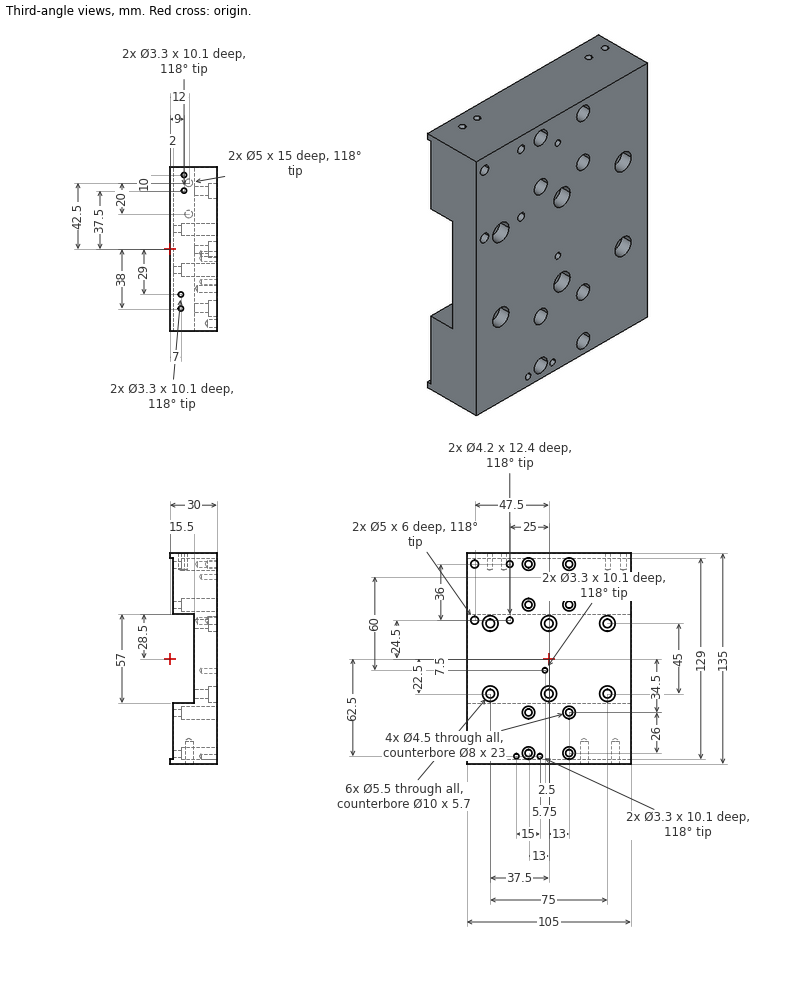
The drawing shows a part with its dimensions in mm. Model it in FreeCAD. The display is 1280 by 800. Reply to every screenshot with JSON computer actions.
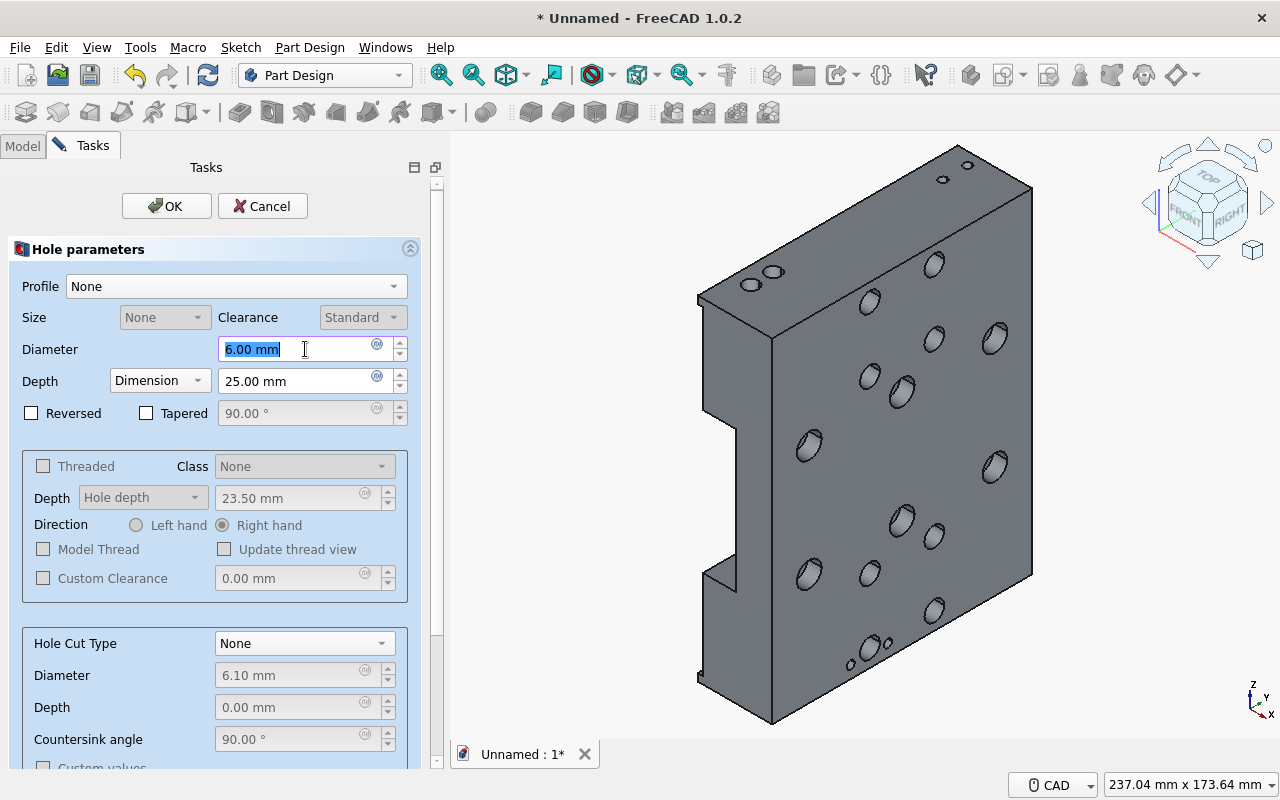
{"action": "type", "text": "3.3"}
{"action": "key", "text": "Tab"}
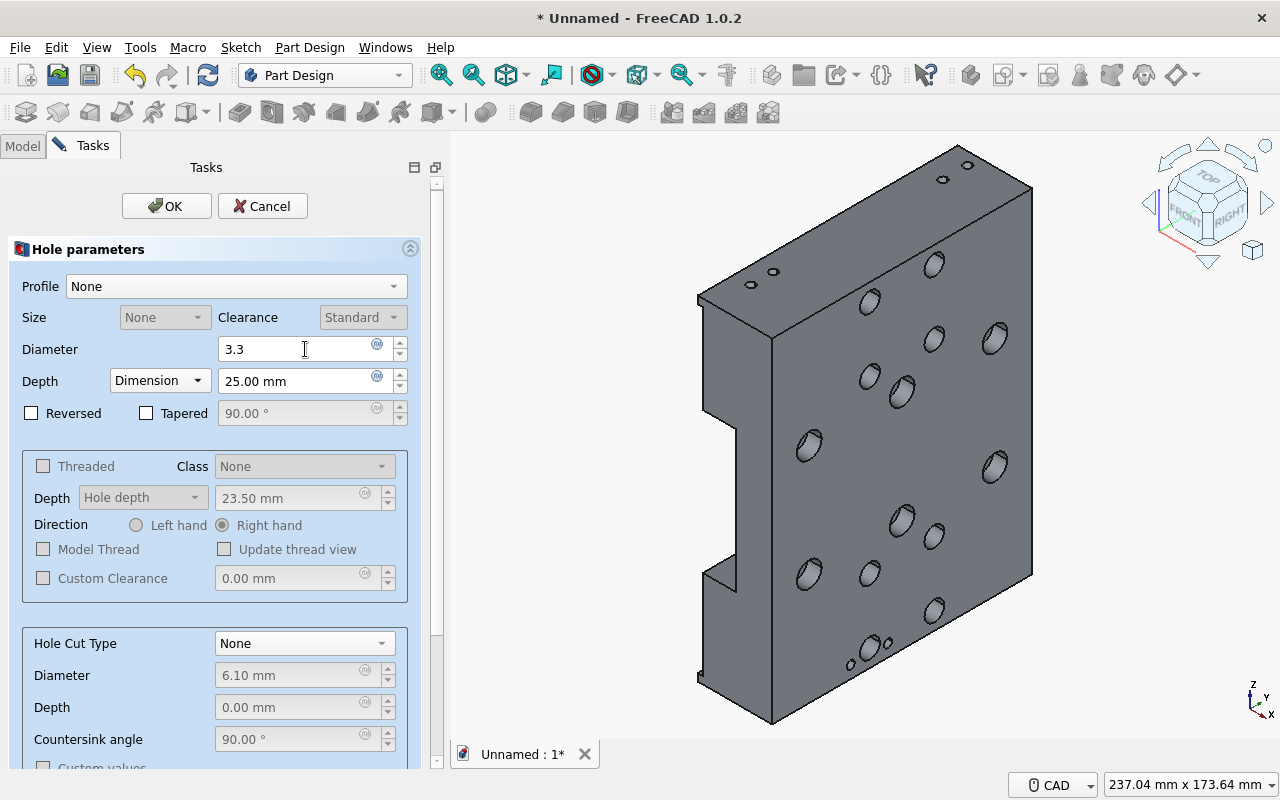
{"action": "triple_click", "coordinate": [305, 381]}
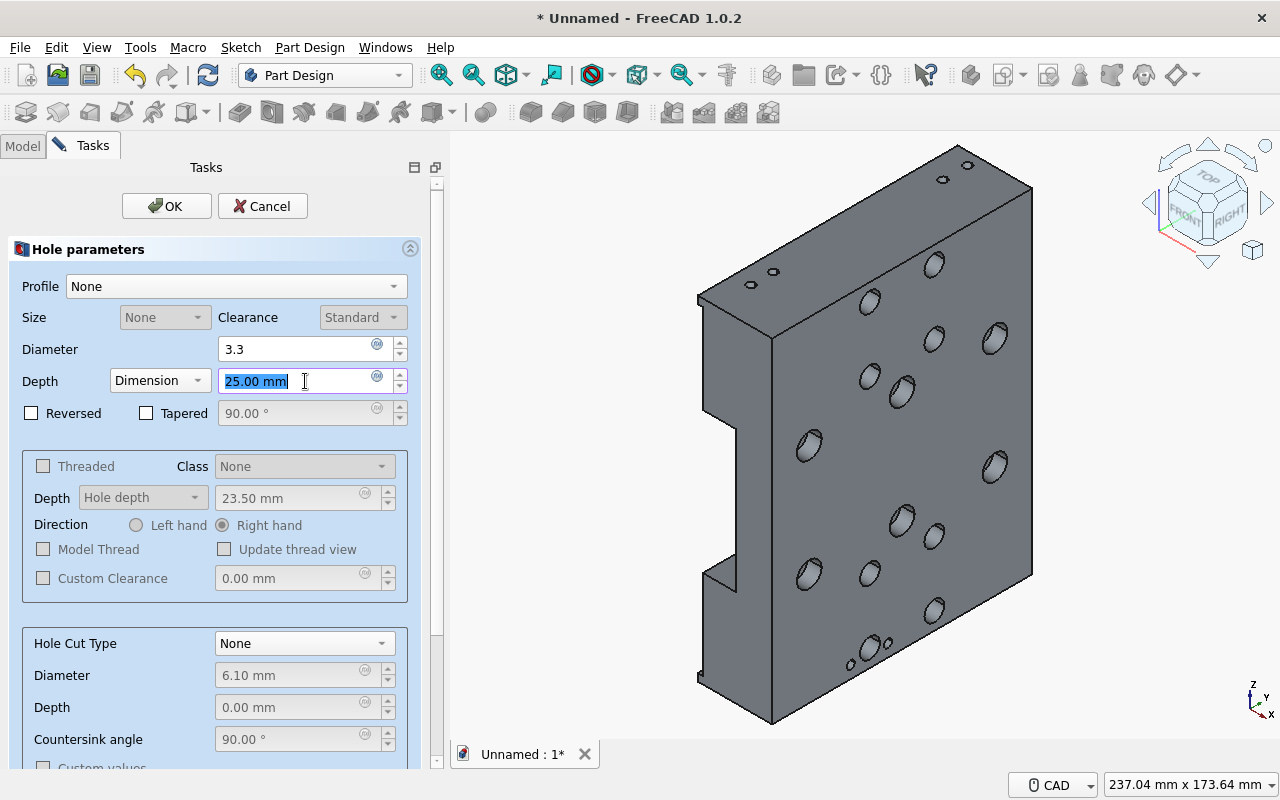
{"action": "type", "text": "10.1"}
{"action": "key", "text": "Tab"}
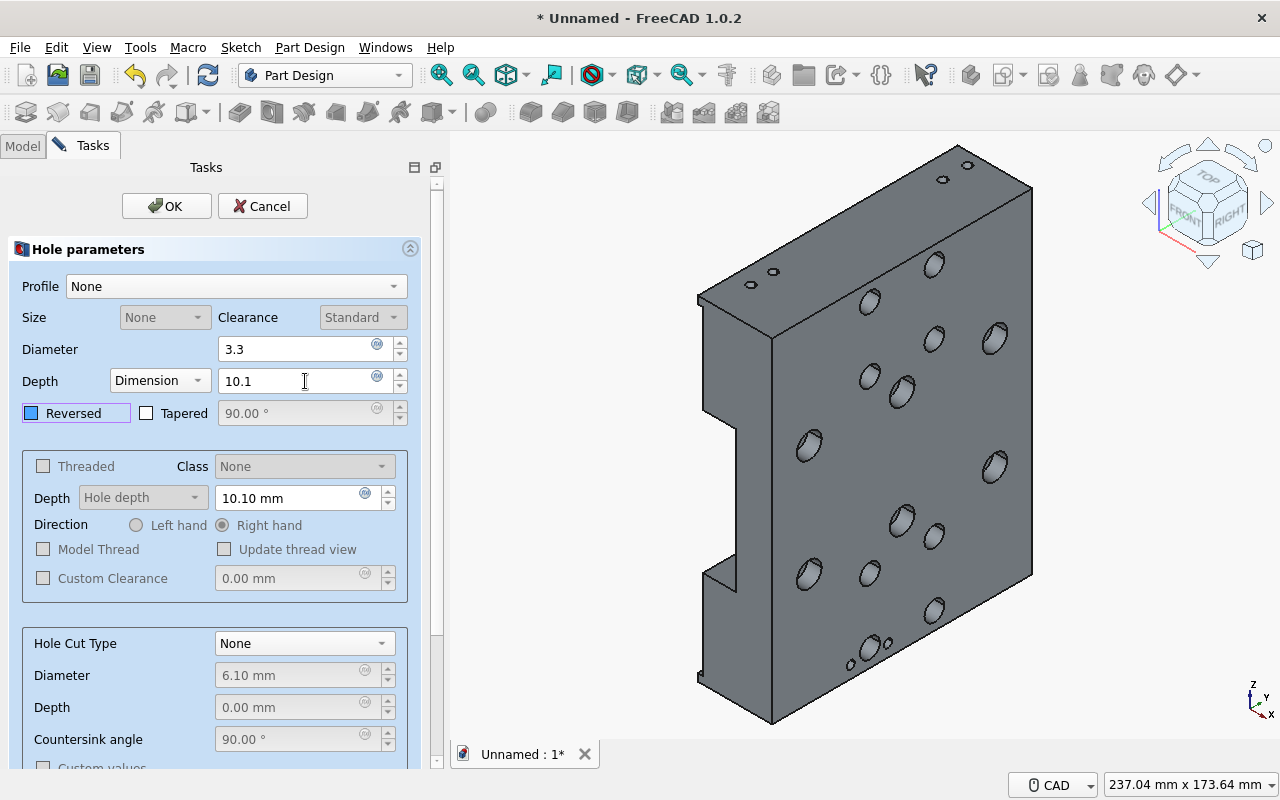
{"action": "left_click", "coordinate": [167, 206]}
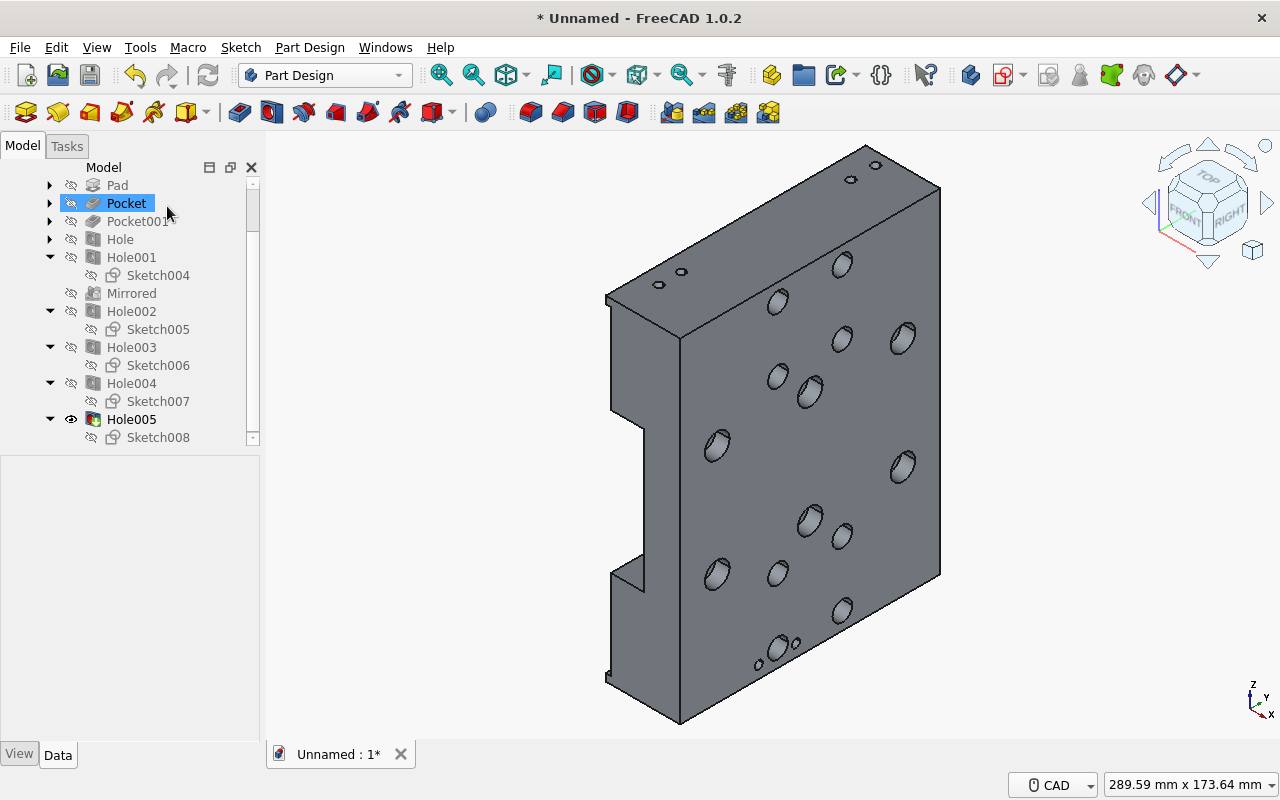
{"action": "left_click", "coordinate": [773, 477]}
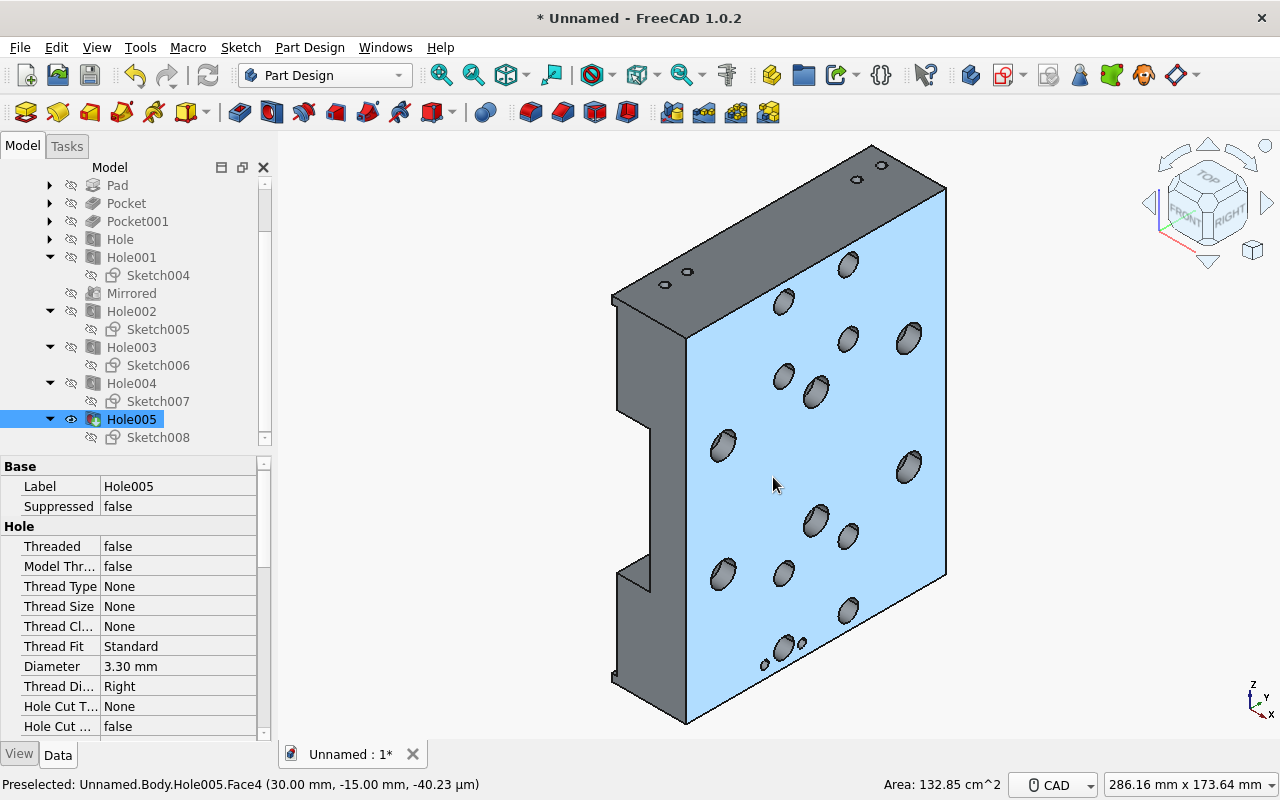
{"action": "left_click", "coordinate": [1004, 76]}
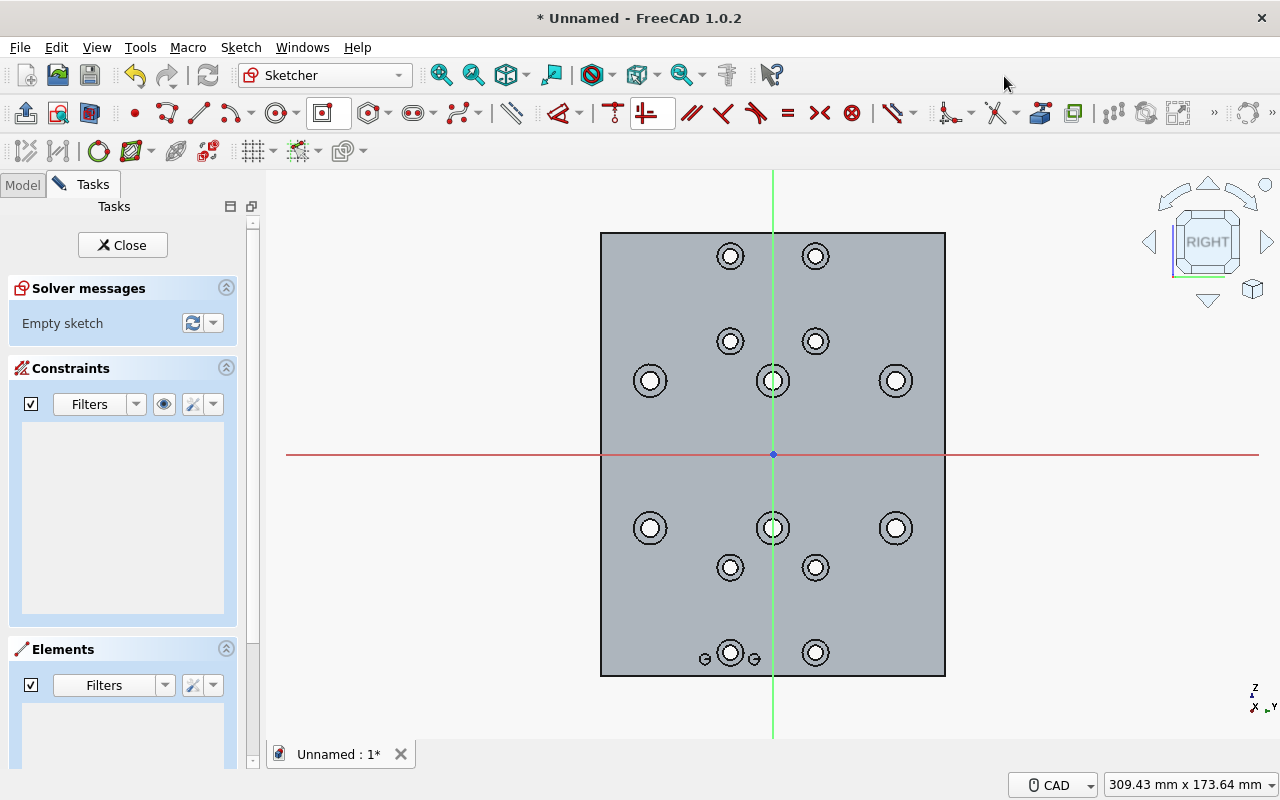
{"action": "scroll", "coordinate": [758, 227], "scroll_direction": "up", "scroll_amount": 3}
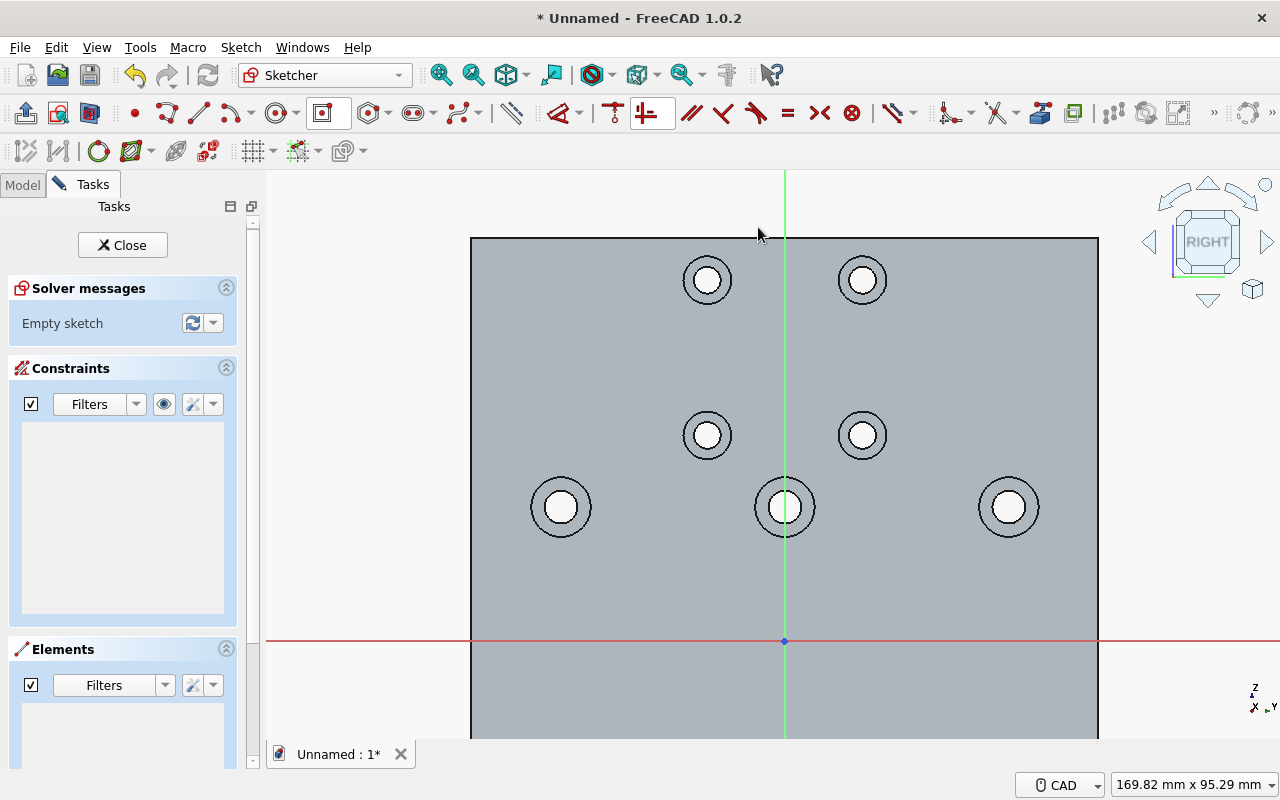
{"action": "left_click", "coordinate": [276, 114]}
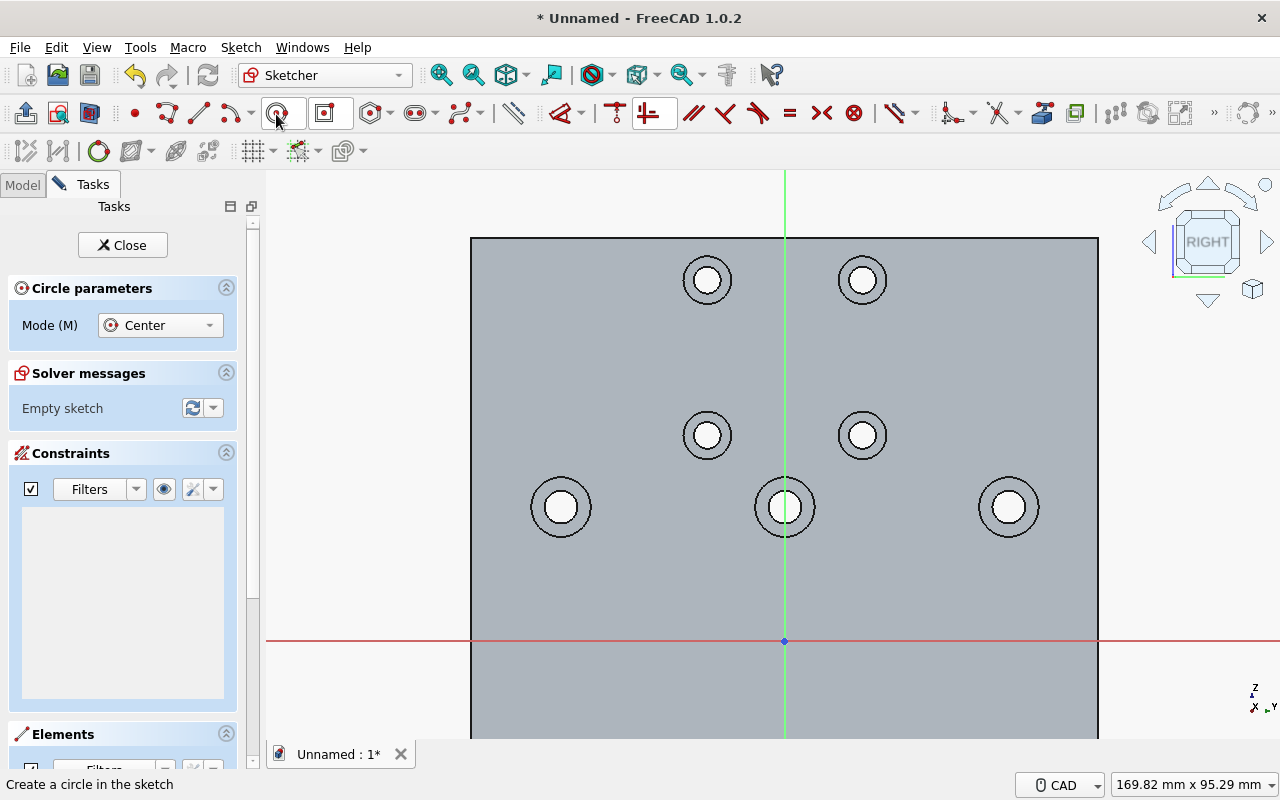
{"action": "scroll", "coordinate": [636, 495], "scroll_direction": "up", "scroll_amount": 3}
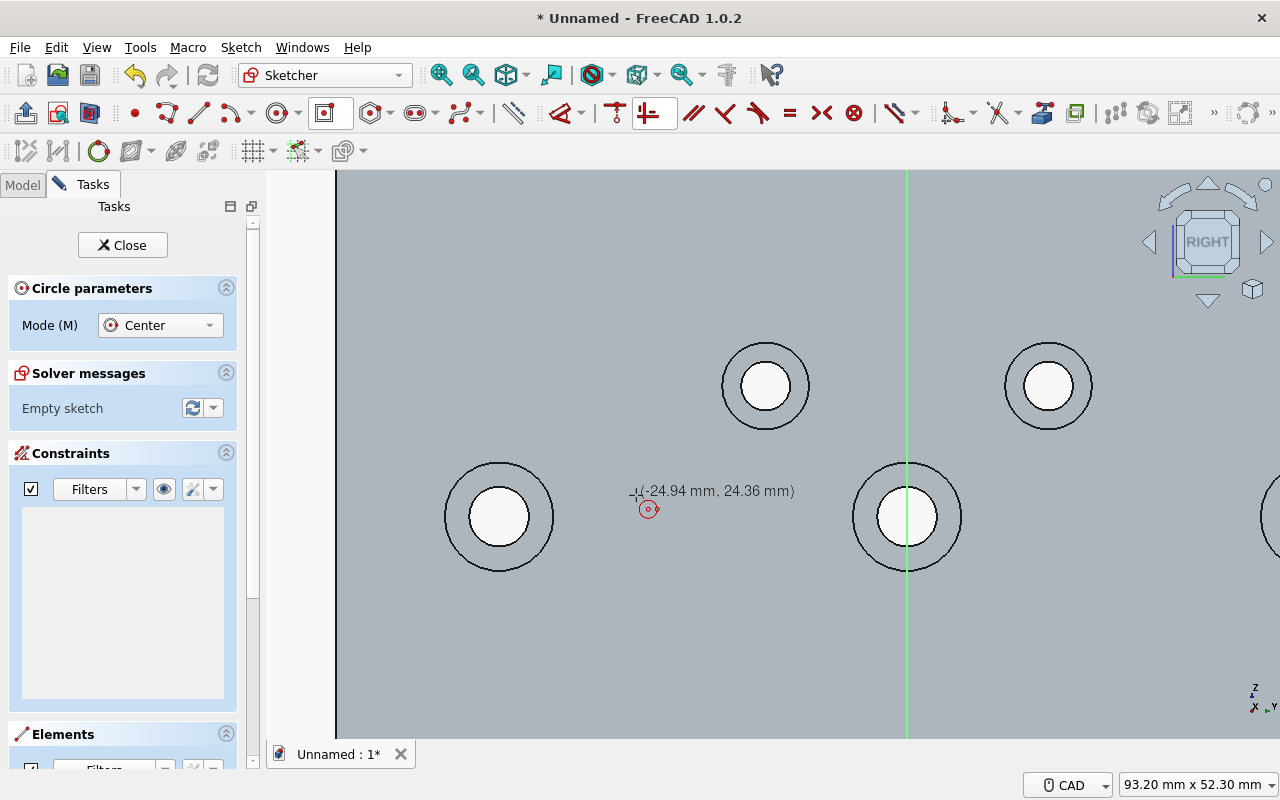
{"action": "left_click", "coordinate": [635, 495]}
{"action": "left_click", "coordinate": [651, 479]}